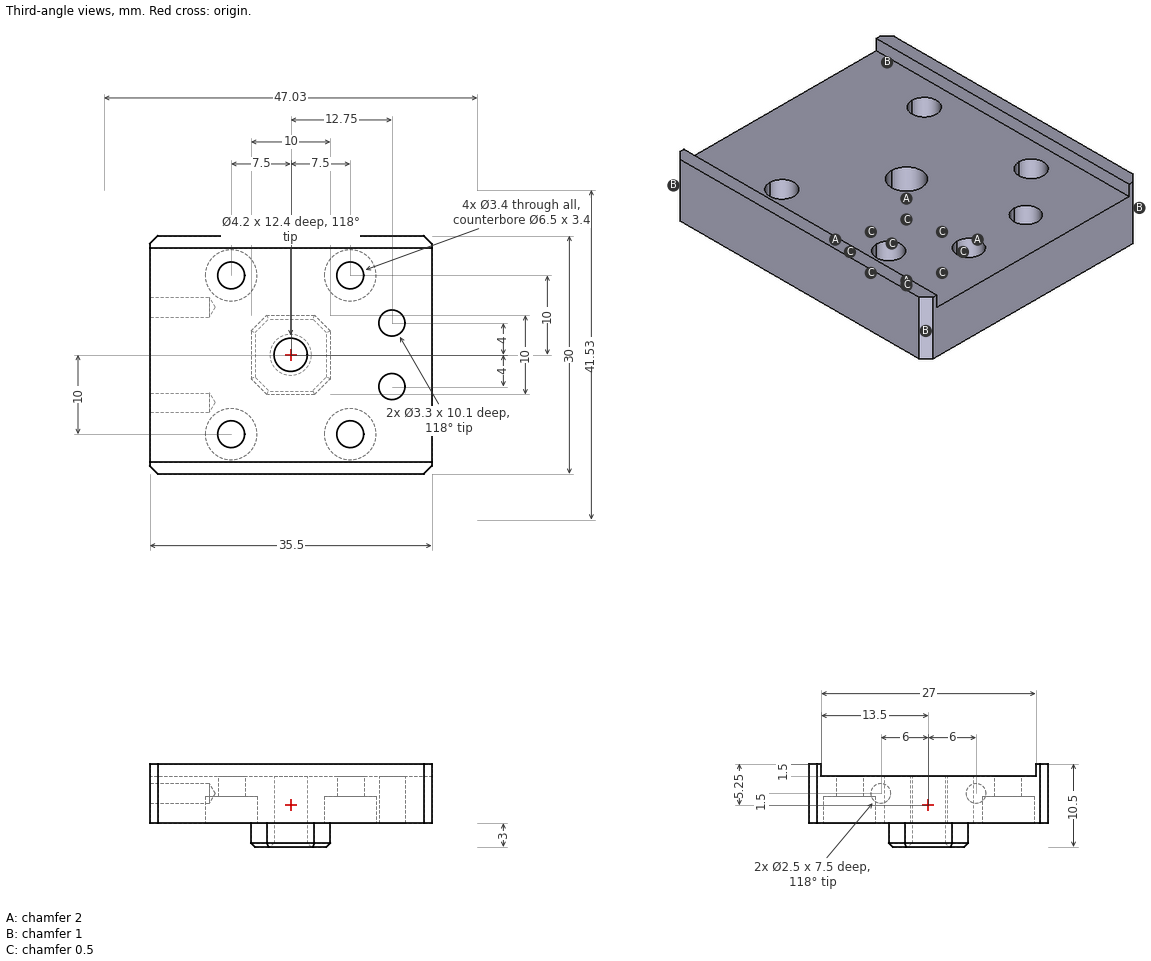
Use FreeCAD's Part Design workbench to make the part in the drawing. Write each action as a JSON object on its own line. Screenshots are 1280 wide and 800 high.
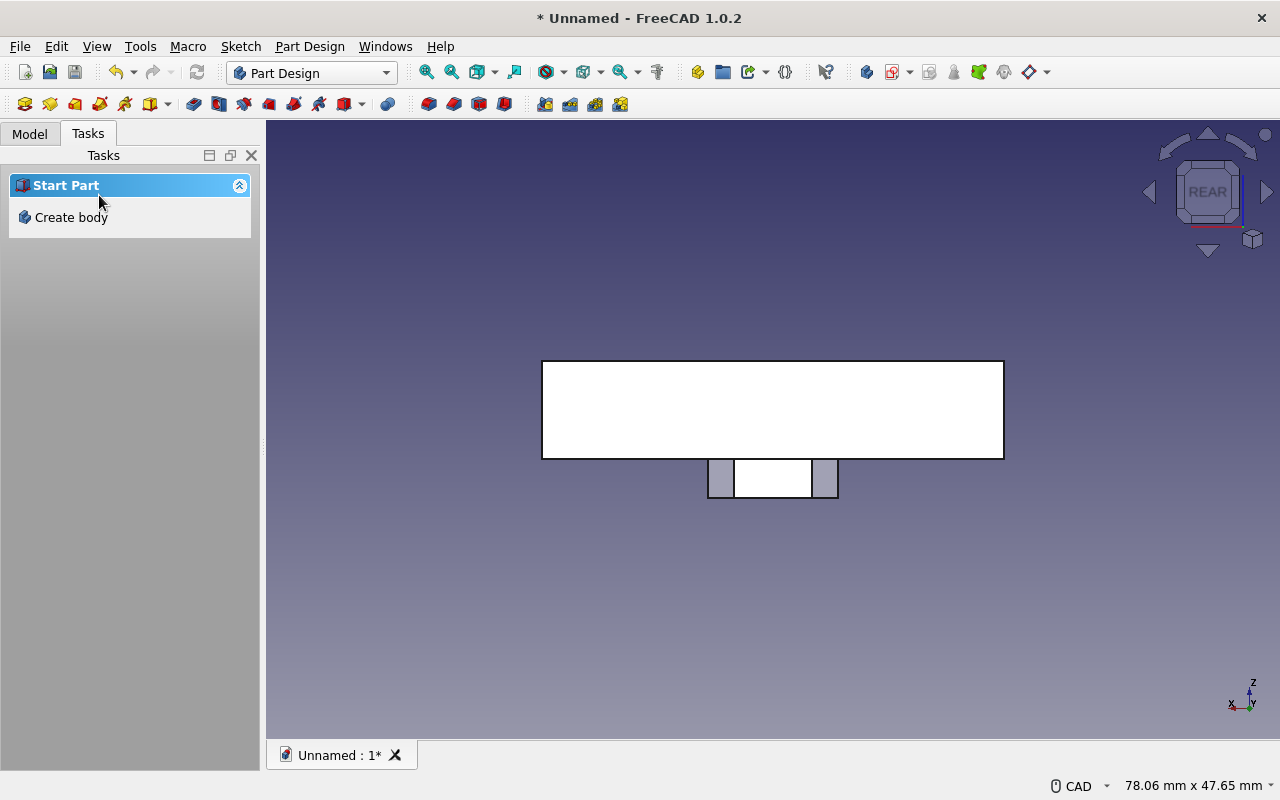
{"action": "key", "text": "5"}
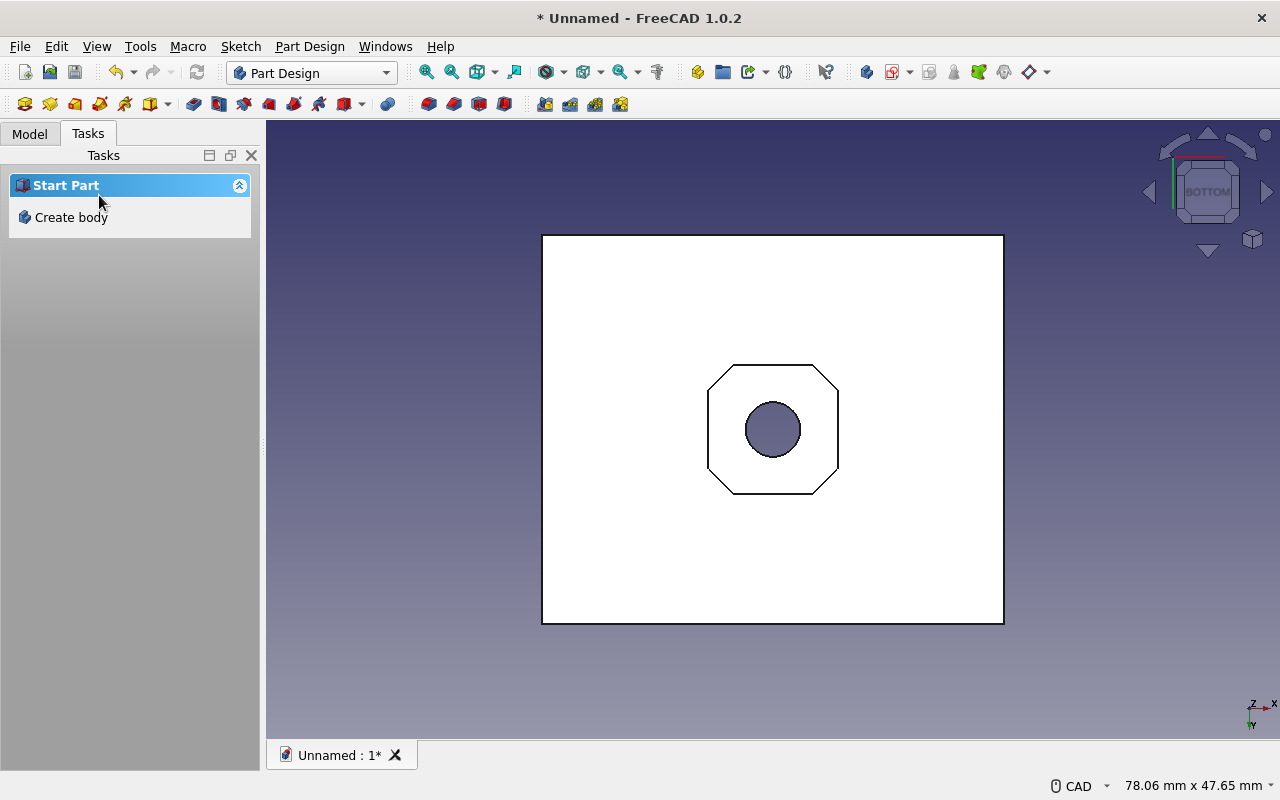
{"action": "left_click", "coordinate": [905, 317]}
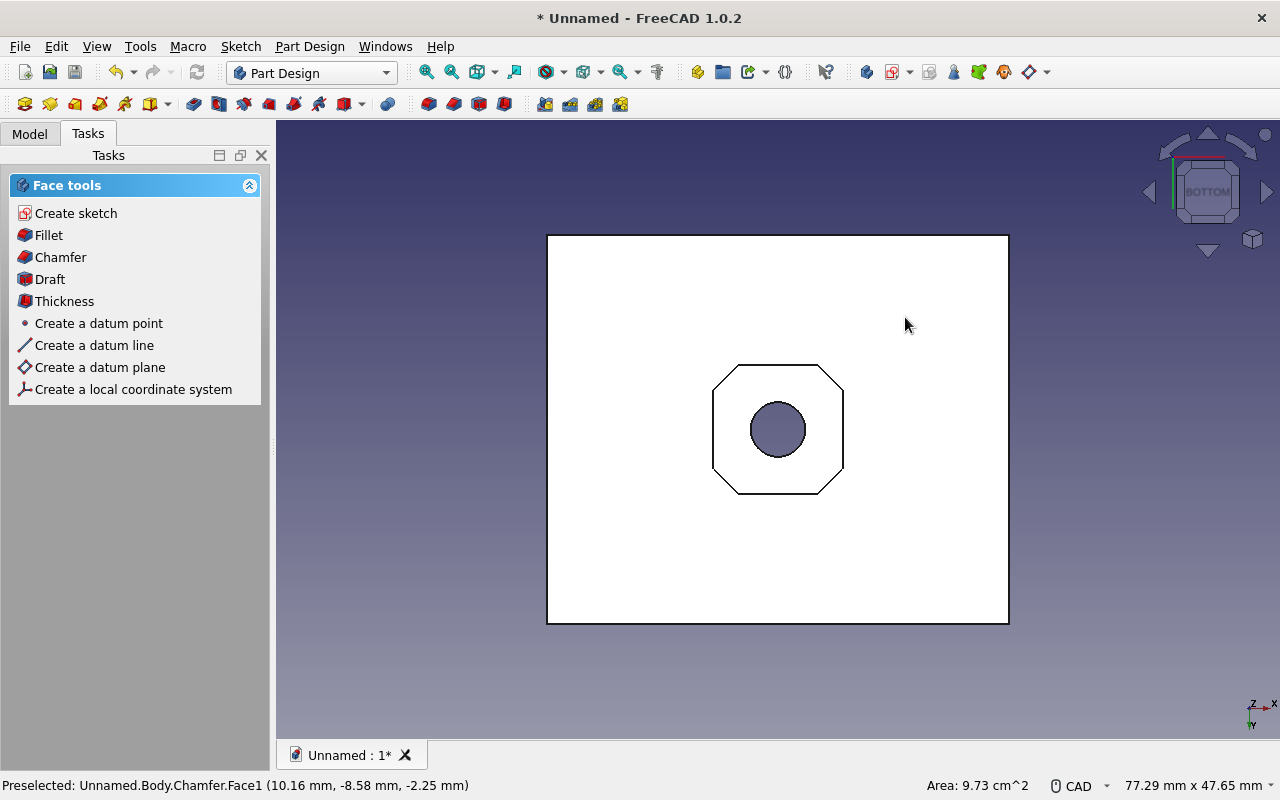
{"action": "left_click", "coordinate": [892, 72]}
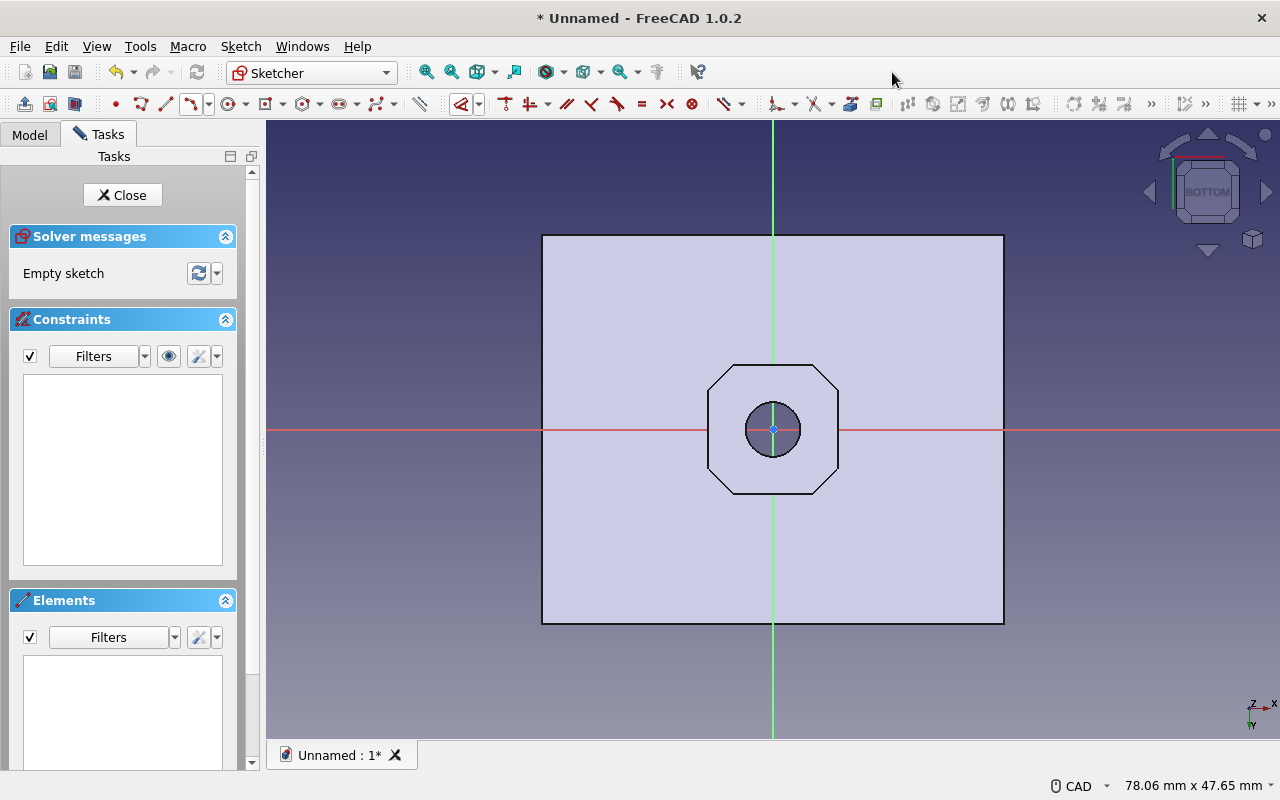
{"action": "scroll", "coordinate": [961, 429], "scroll_direction": "up", "scroll_amount": 5}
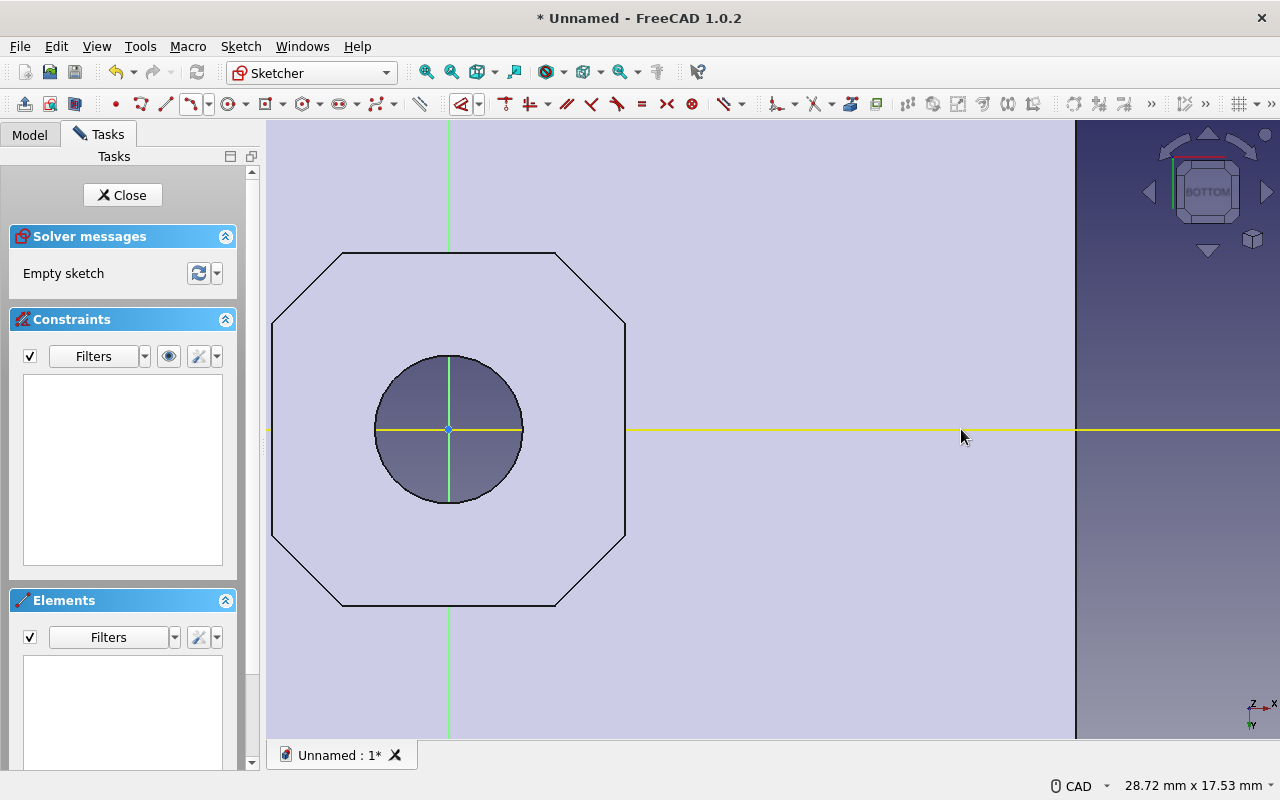
{"action": "left_click", "coordinate": [228, 104]}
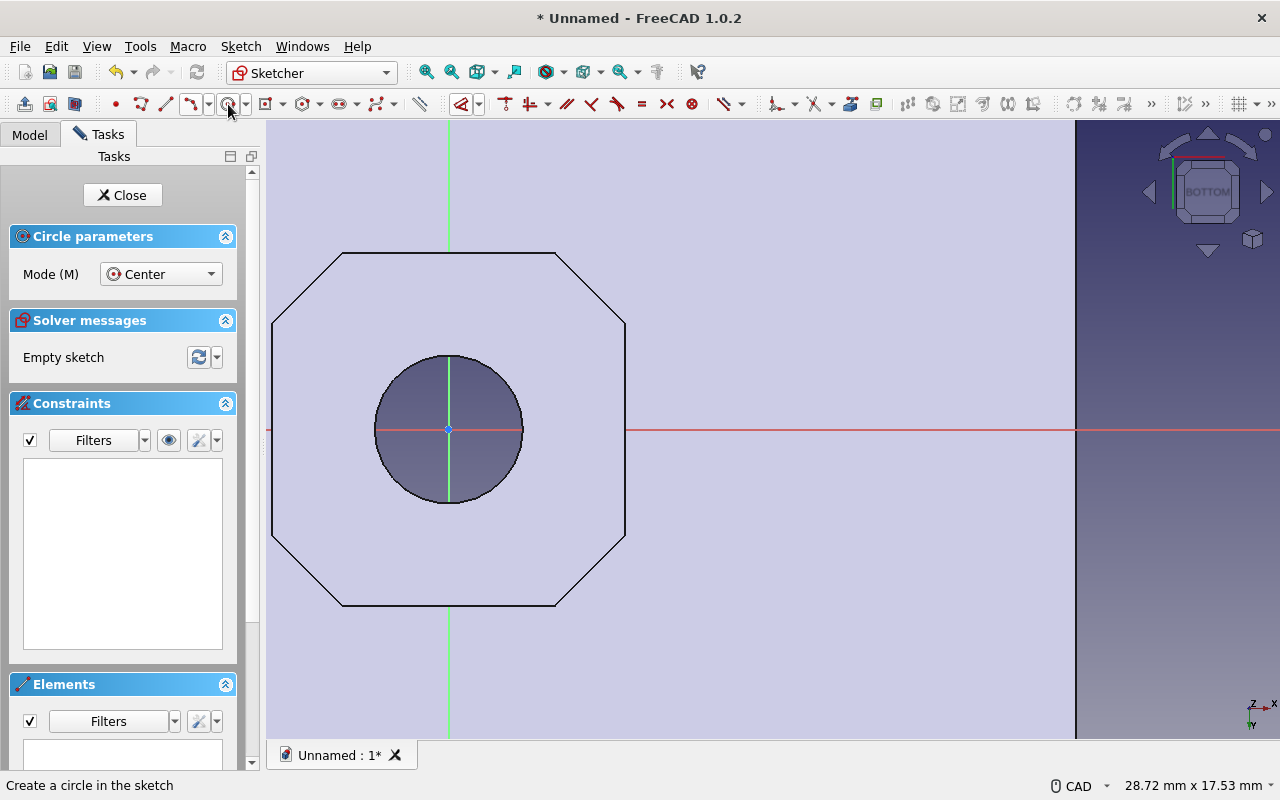
{"action": "left_click", "coordinate": [899, 571]}
{"action": "left_click", "coordinate": [940, 530]}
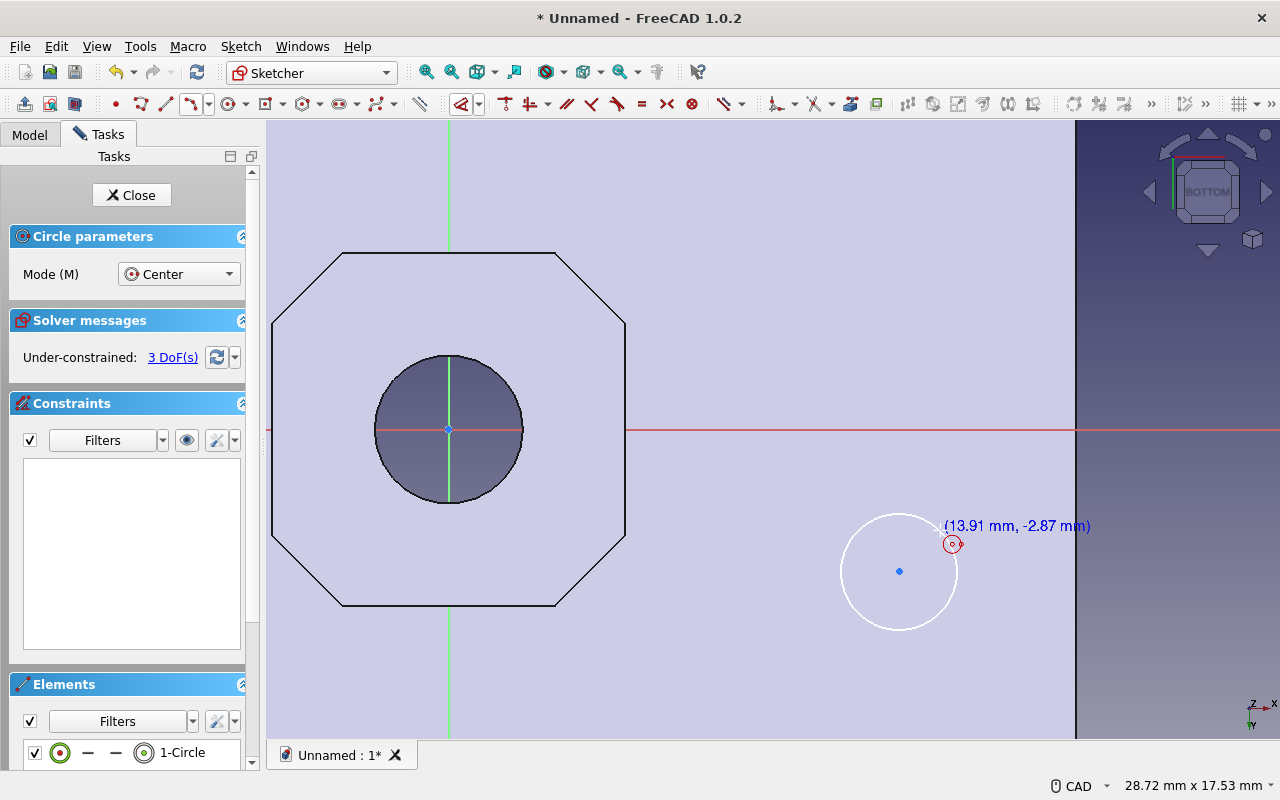
{"action": "left_click", "coordinate": [899, 288]}
{"action": "left_click", "coordinate": [940, 247]}
{"action": "key", "text": "Escape"}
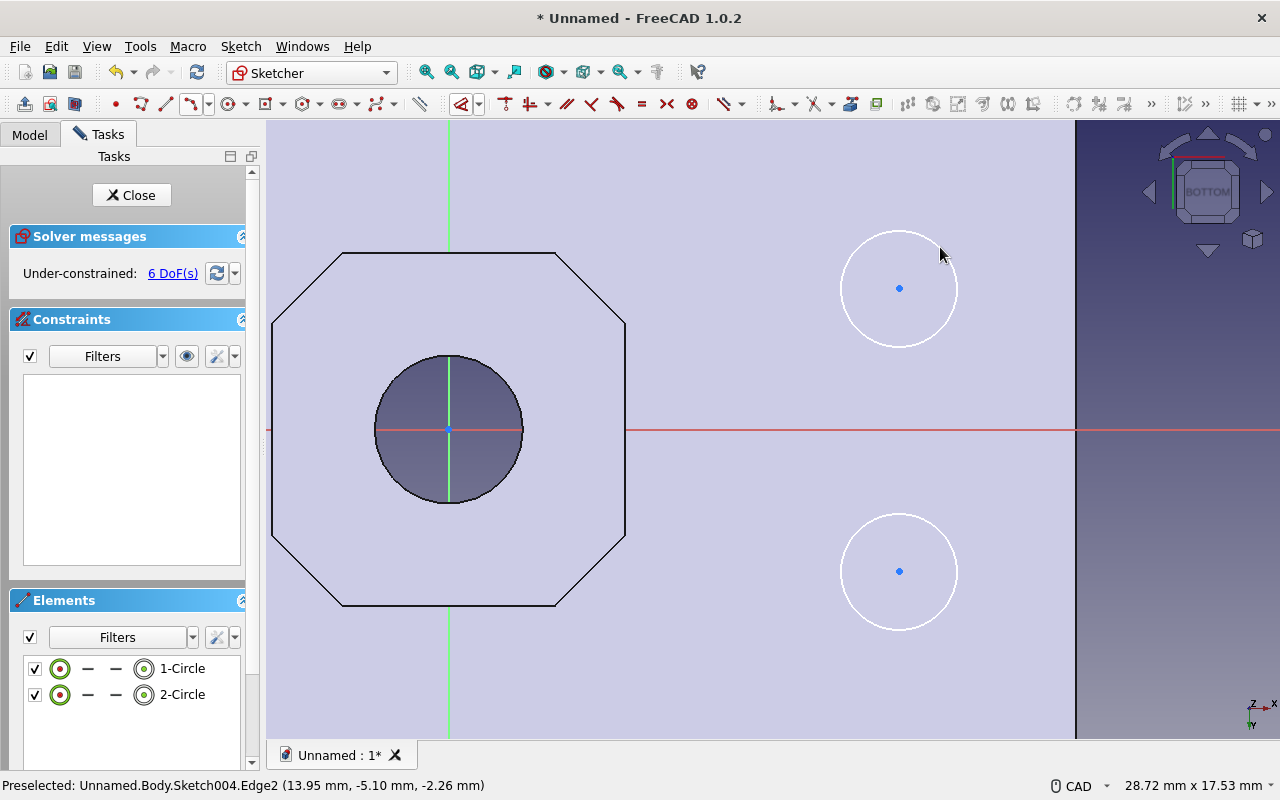
{"action": "left_click", "coordinate": [940, 531]}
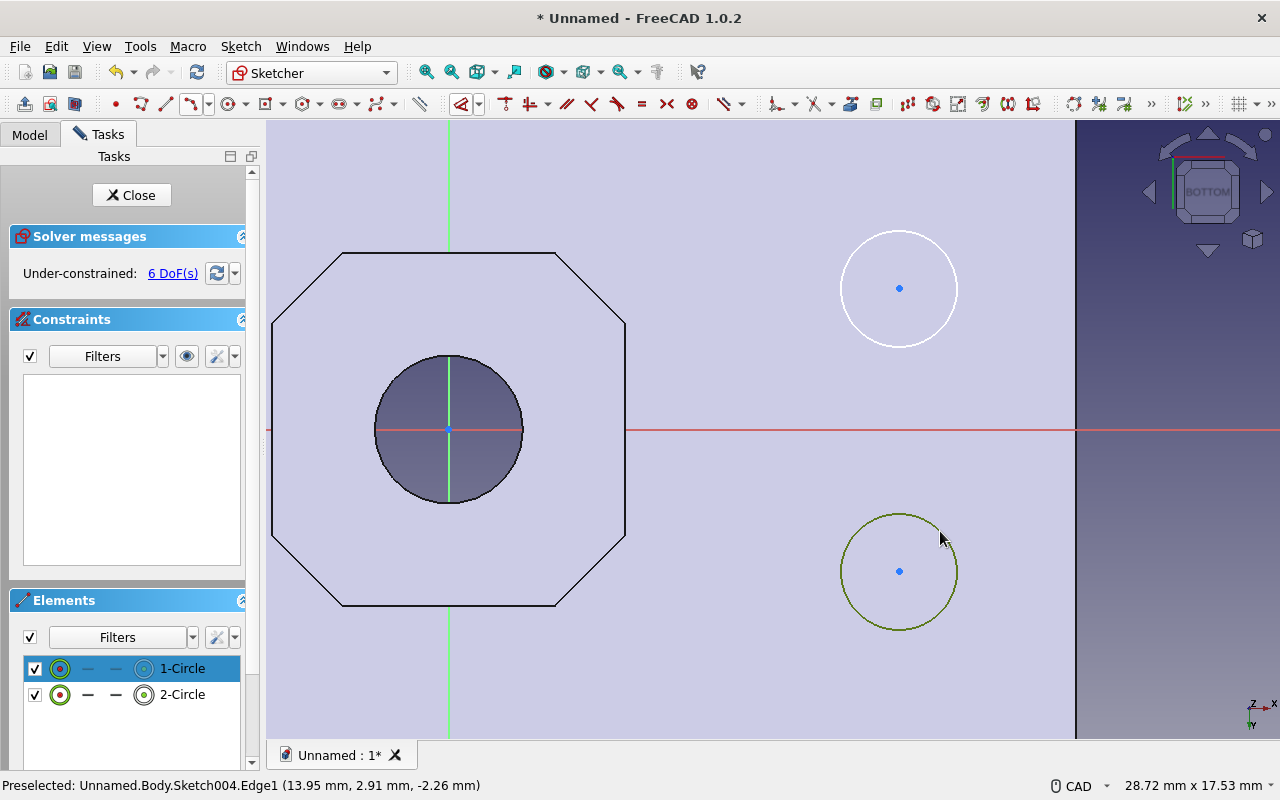
{"action": "left_click", "coordinate": [940, 248]}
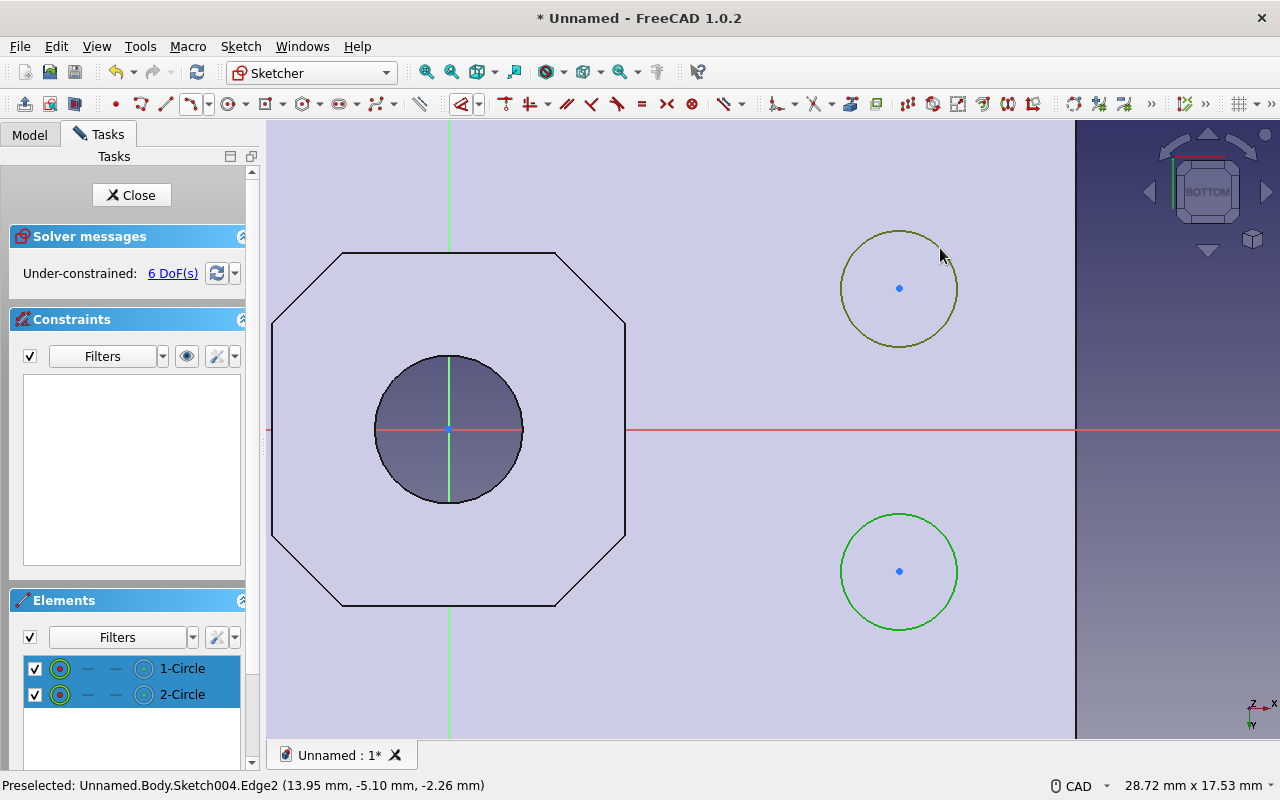
{"action": "key", "text": "e"}